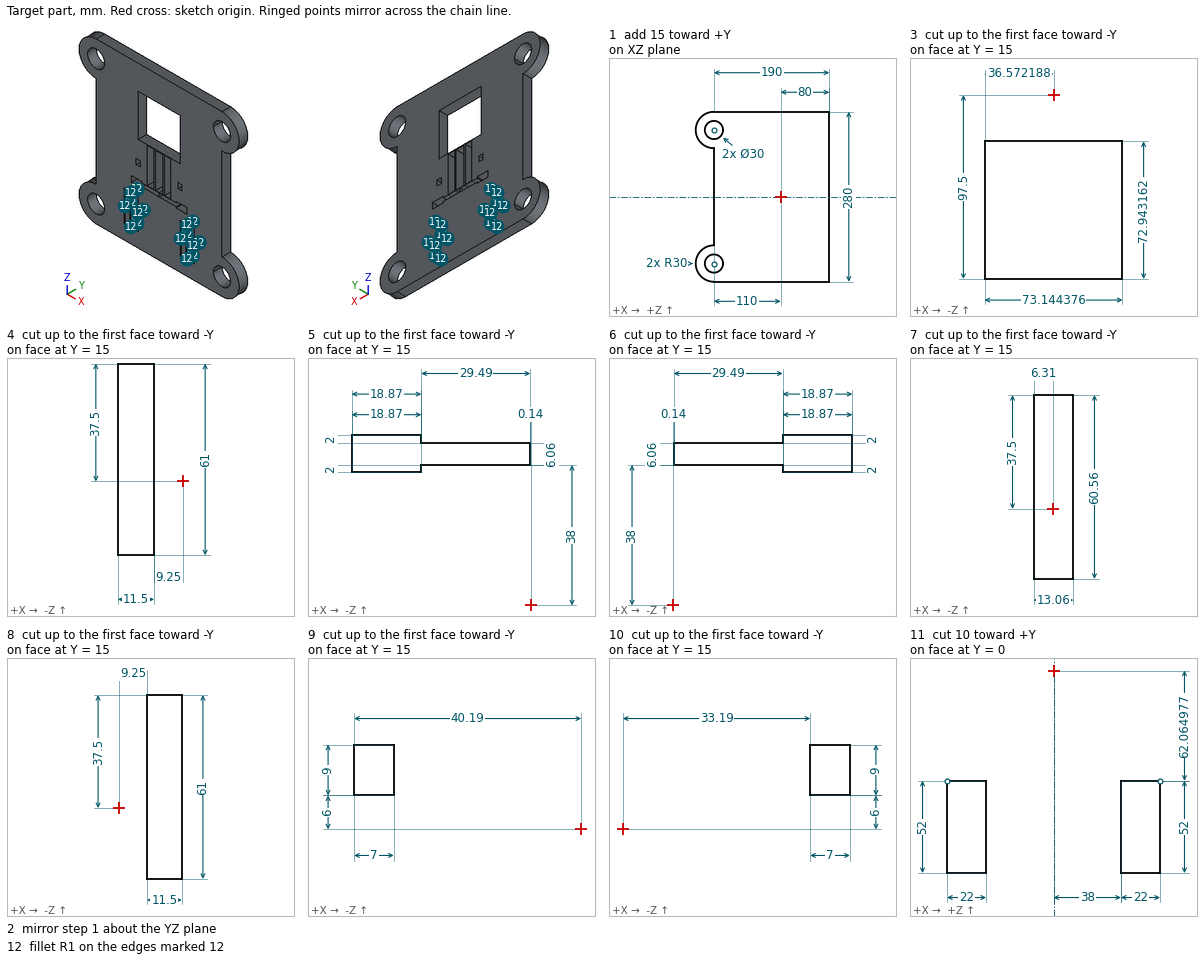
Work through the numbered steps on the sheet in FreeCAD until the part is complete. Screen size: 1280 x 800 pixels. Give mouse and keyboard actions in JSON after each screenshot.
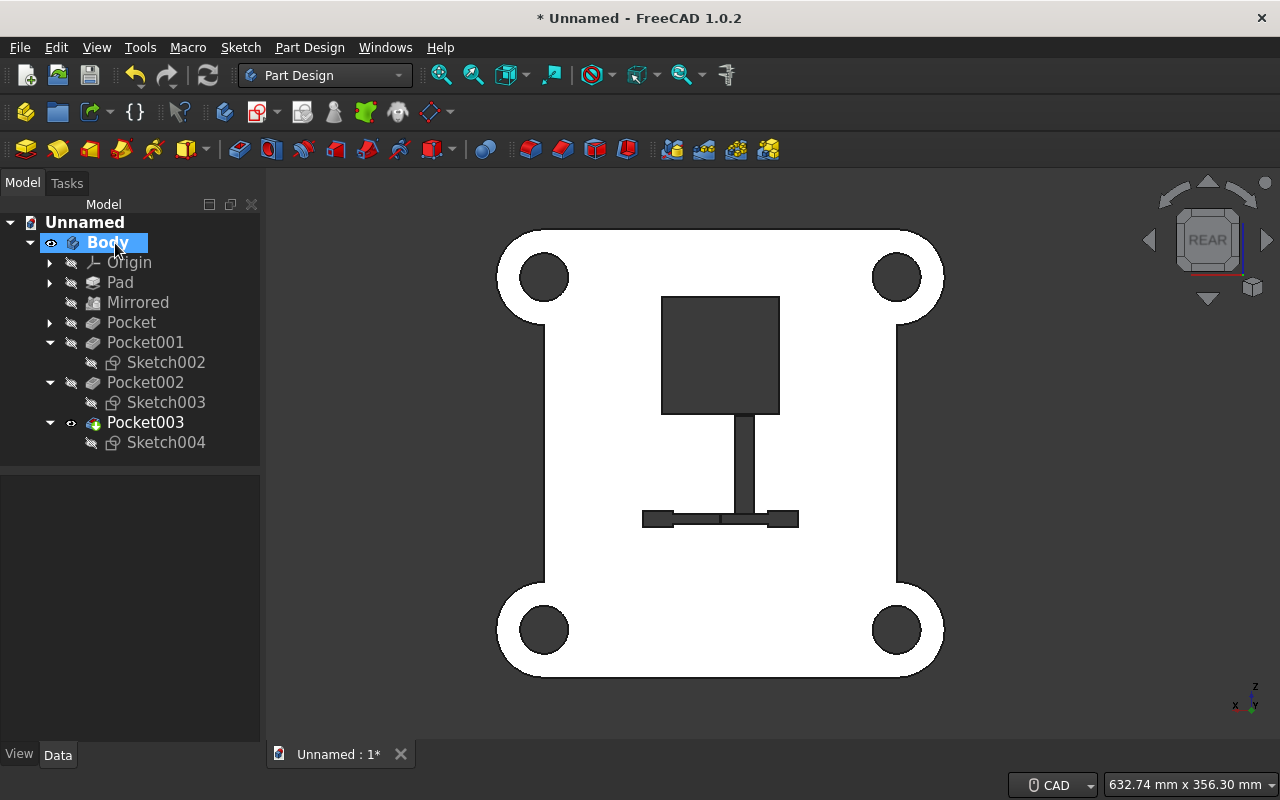
{"action": "left_click", "coordinate": [720, 581]}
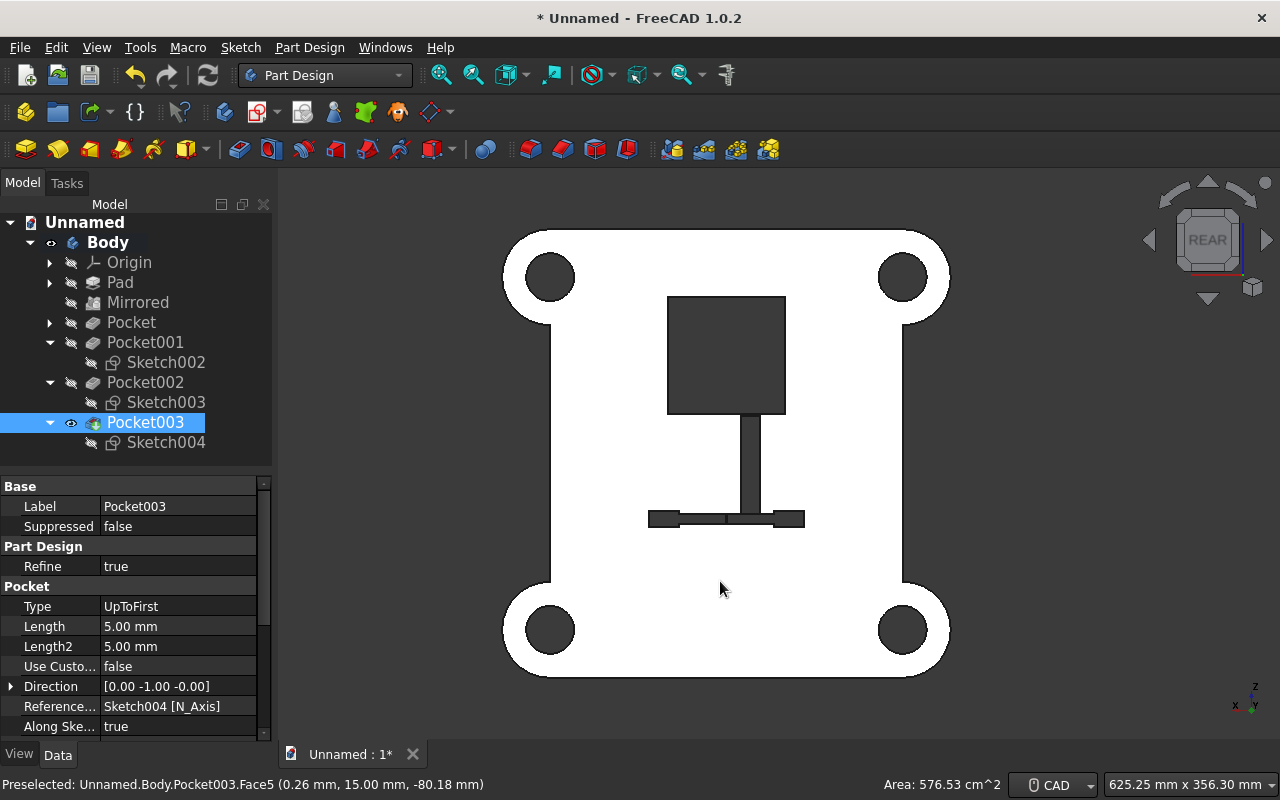
{"action": "left_click", "coordinate": [258, 112]}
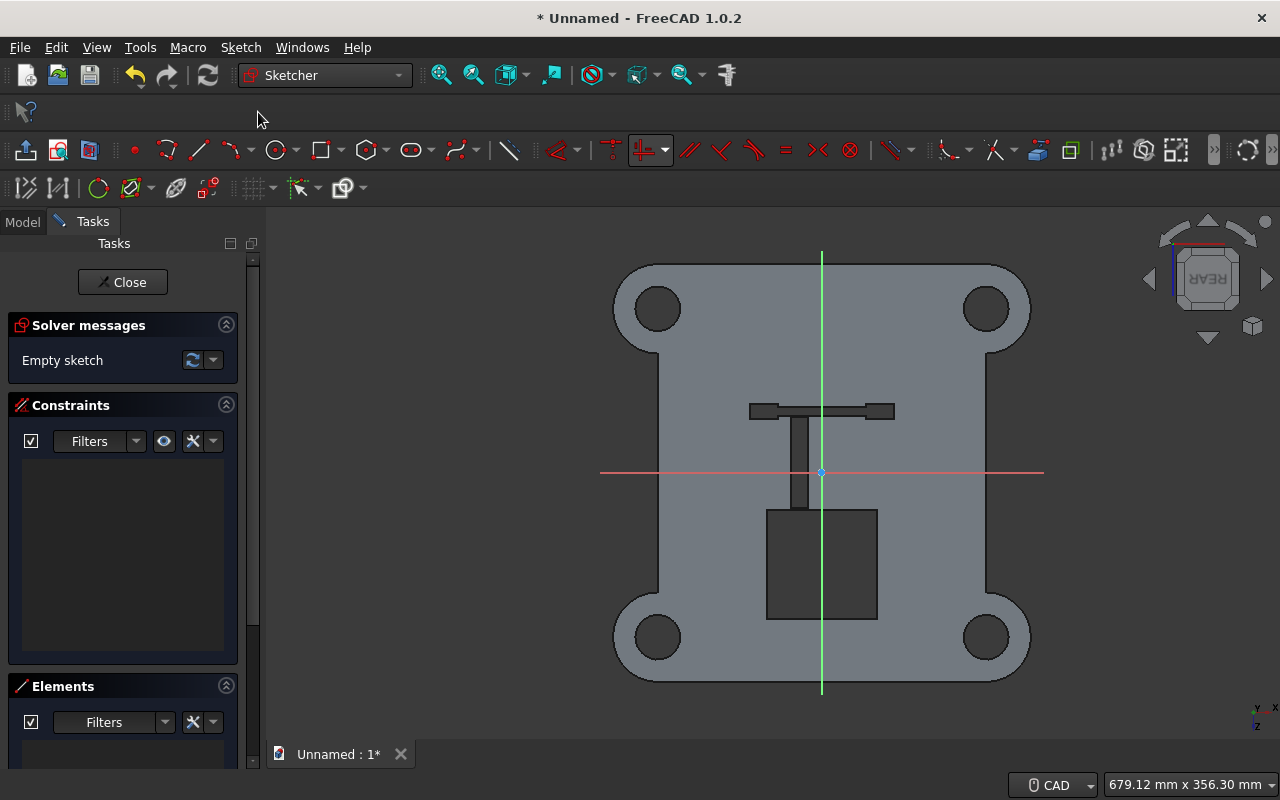
{"action": "scroll", "coordinate": [861, 459], "scroll_direction": "up", "scroll_amount": 7}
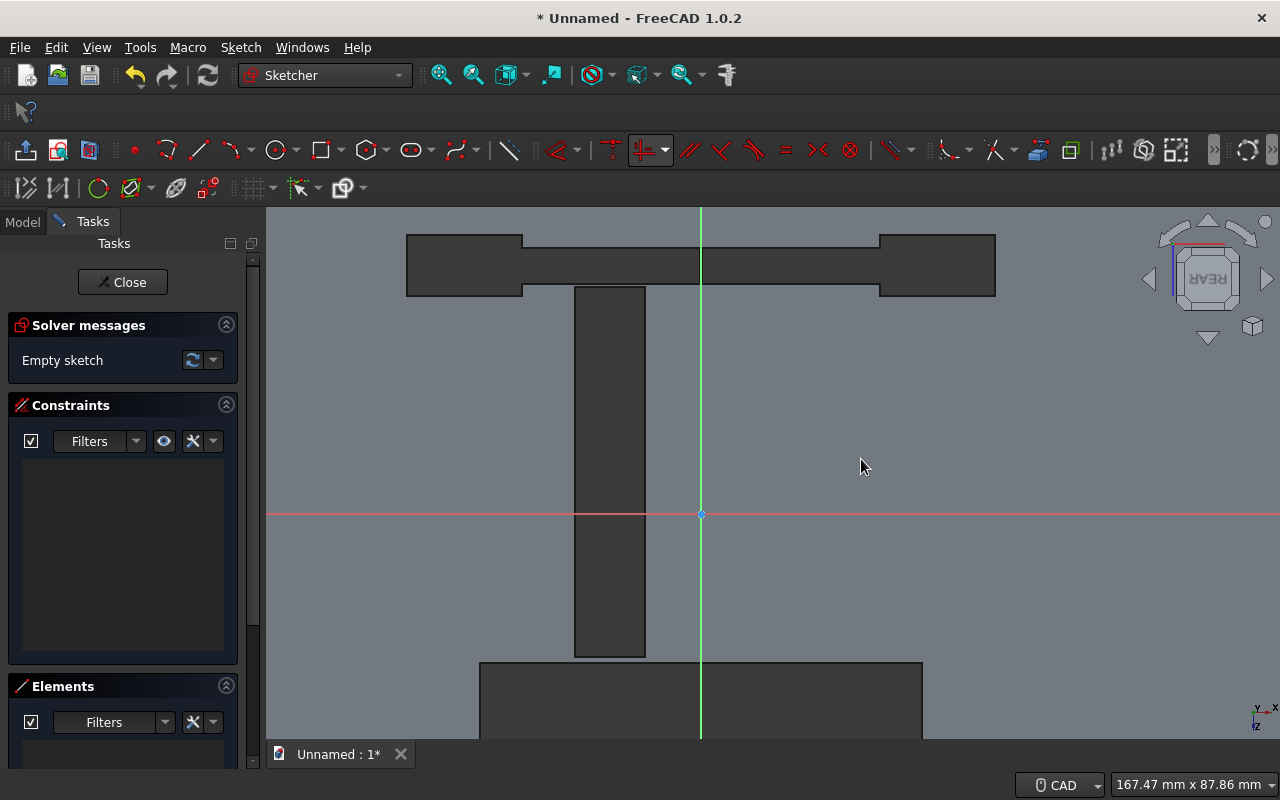
{"action": "left_click", "coordinate": [322, 150]}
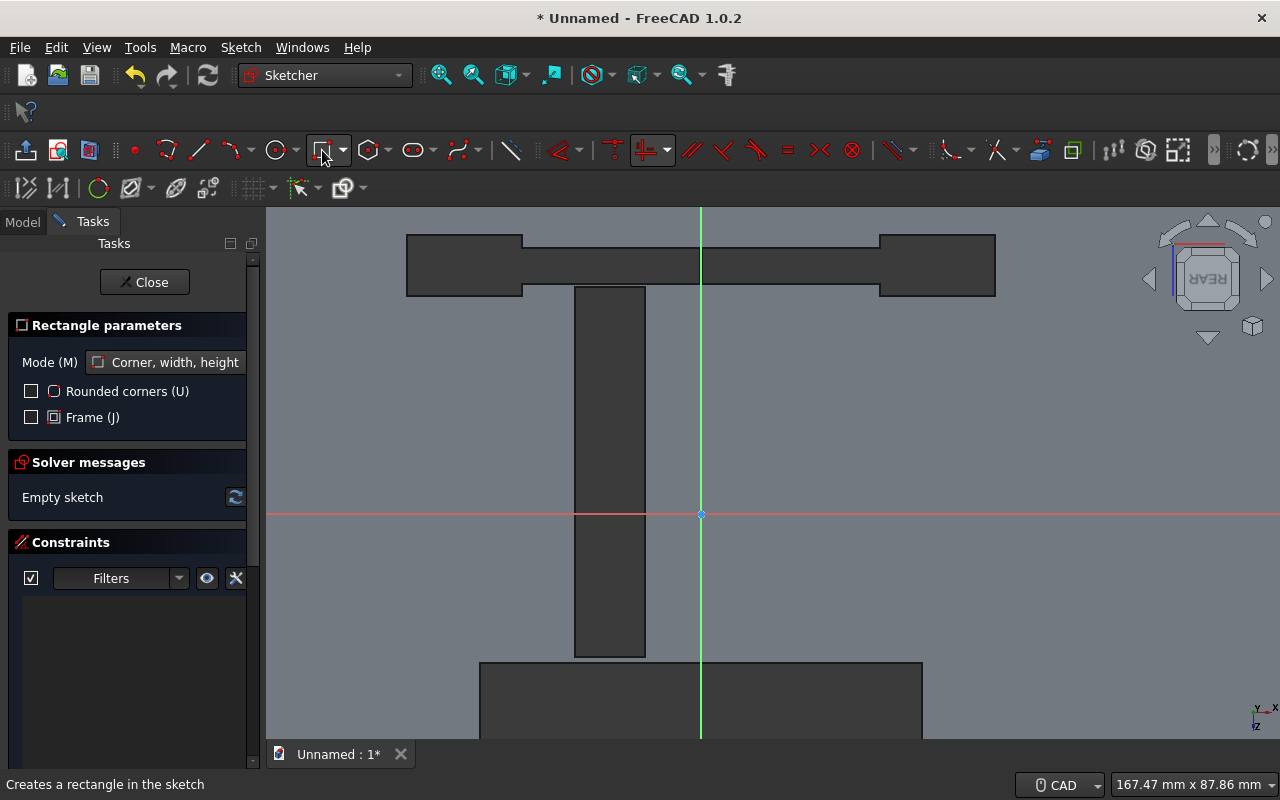
{"action": "left_click", "coordinate": [663, 287]}
{"action": "mouse_move", "coordinate": [742, 654]}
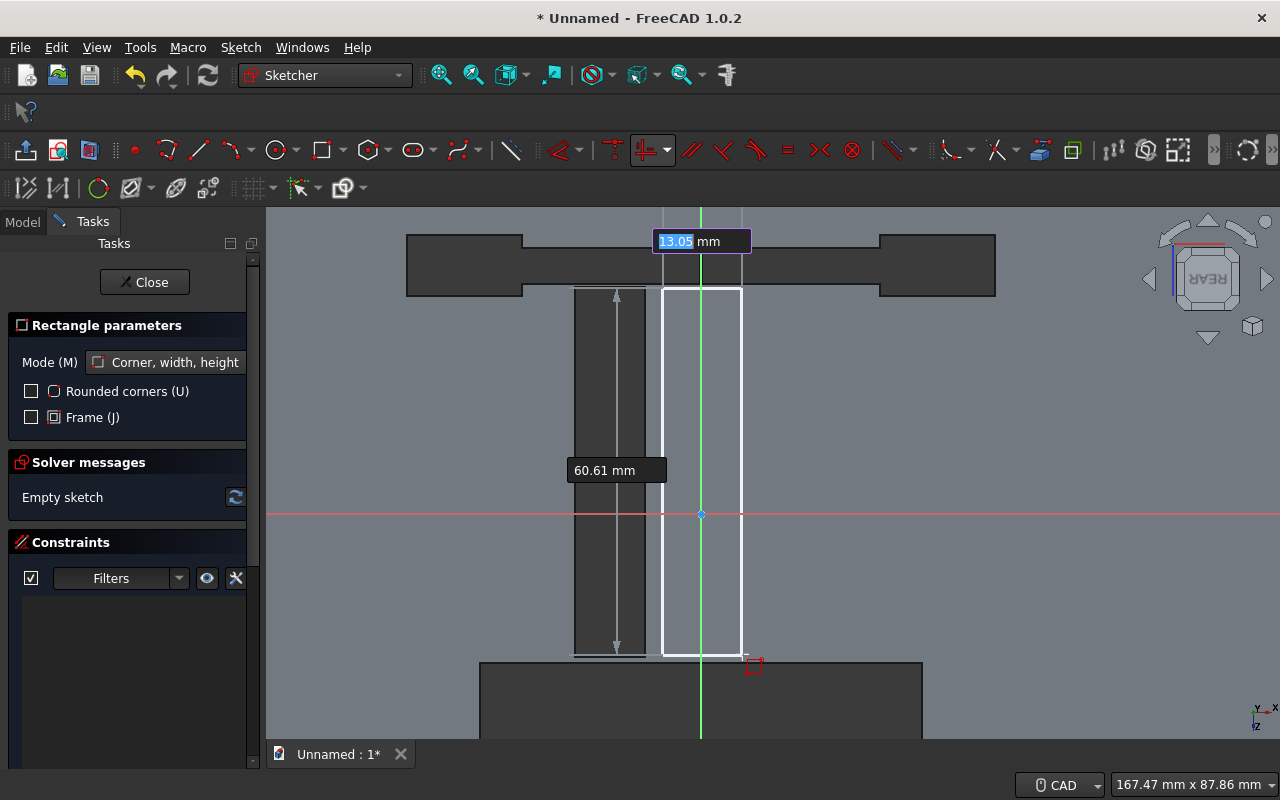
{"action": "type", "text": "13.06"}
{"action": "key", "text": "Tab"}
{"action": "type", "text": "60.56"}
{"action": "key", "text": "Return"}
{"action": "key", "text": "Escape"}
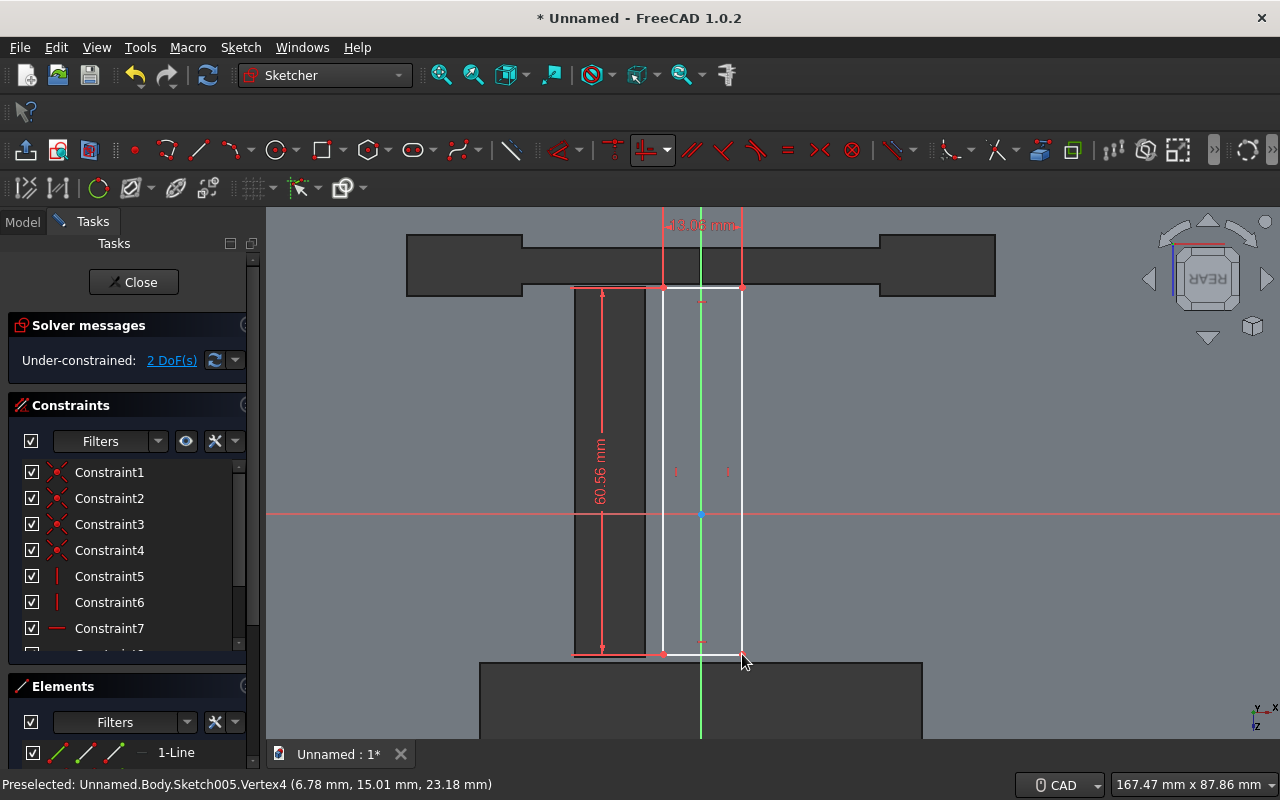
{"action": "key", "text": "d"}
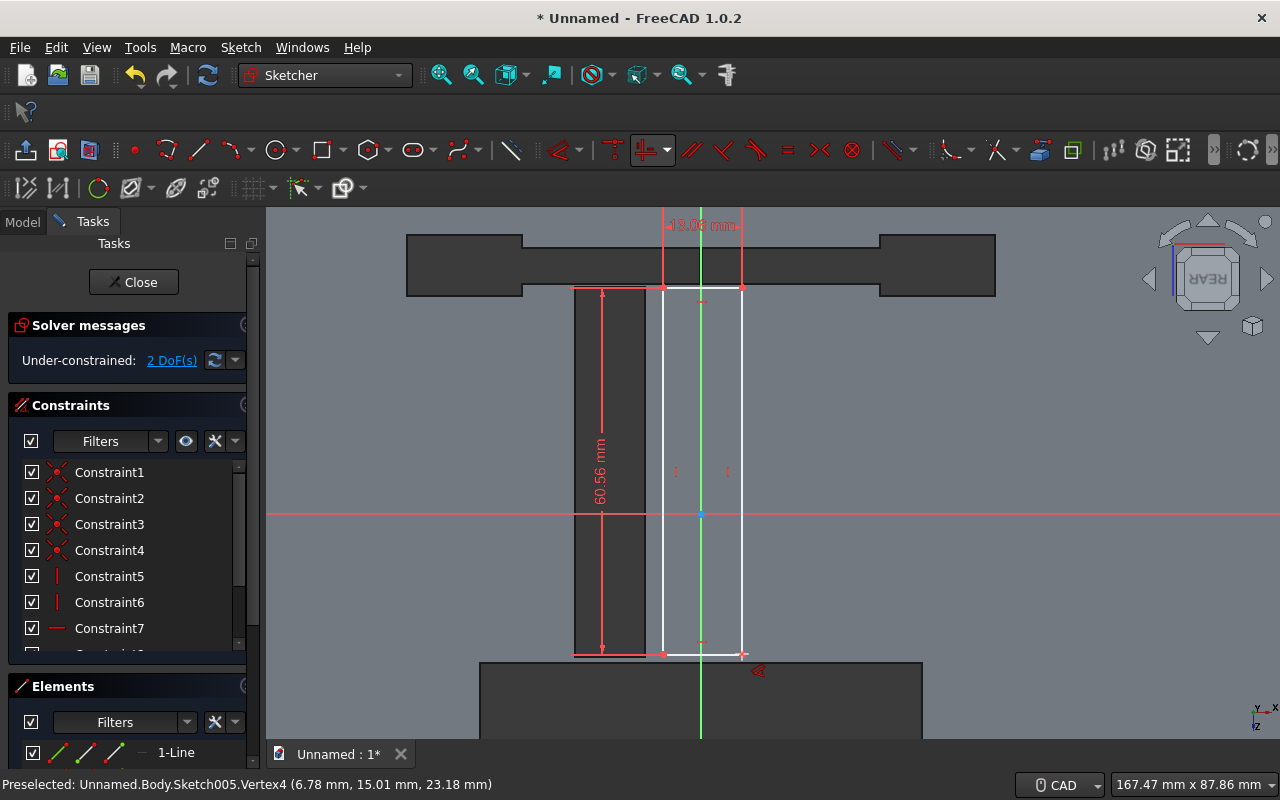
{"action": "left_click", "coordinate": [663, 288]}
{"action": "left_click", "coordinate": [682, 254]}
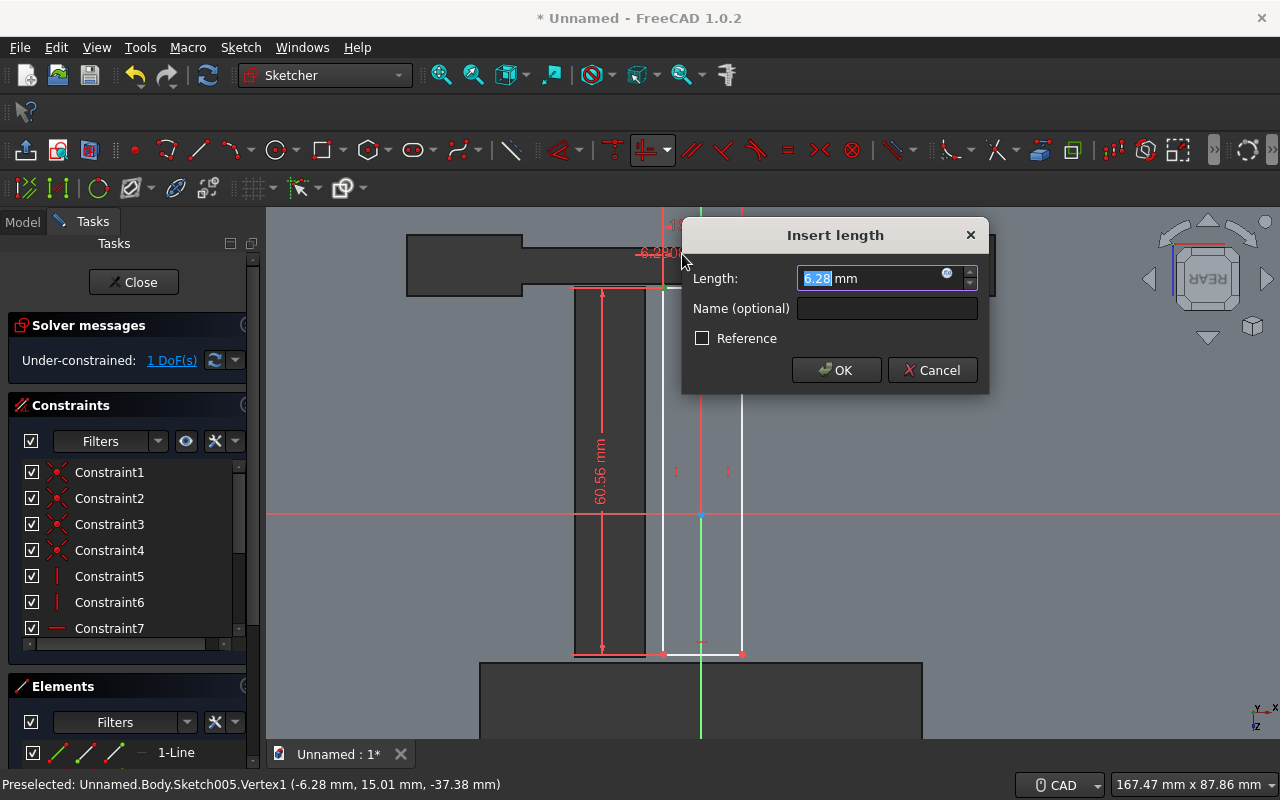
{"action": "type", "text": "6.31"}
{"action": "key", "text": "Return"}